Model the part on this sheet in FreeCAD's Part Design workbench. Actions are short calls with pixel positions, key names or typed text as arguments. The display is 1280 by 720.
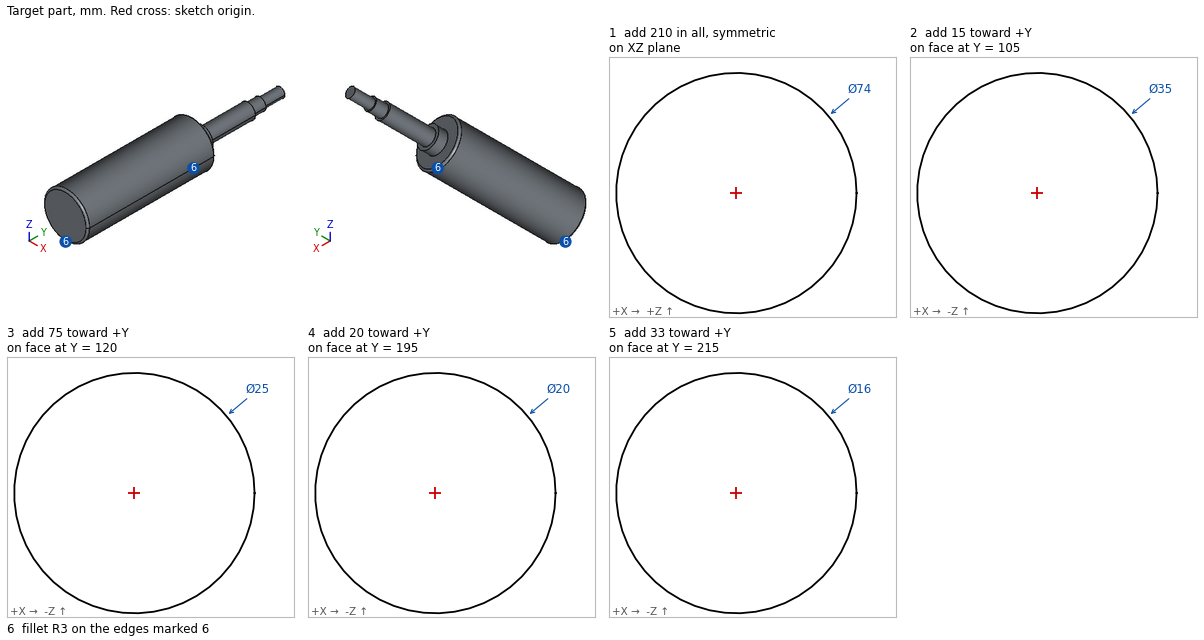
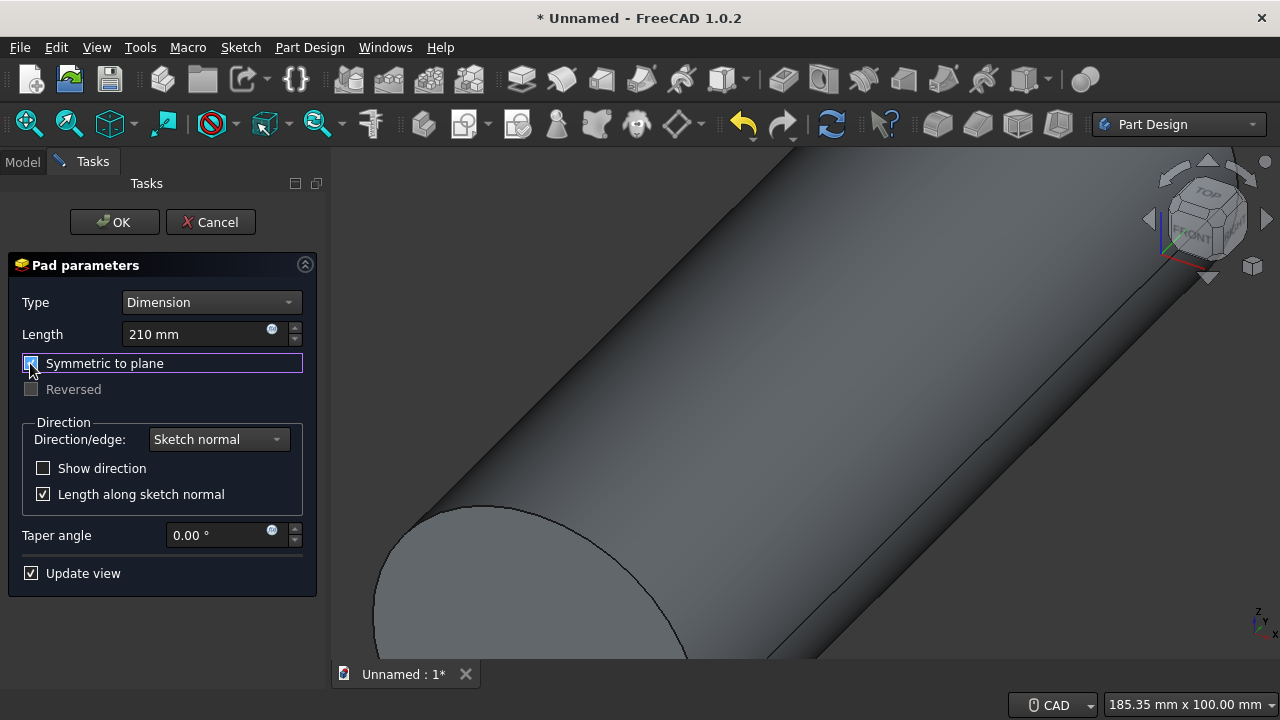
click(115, 222)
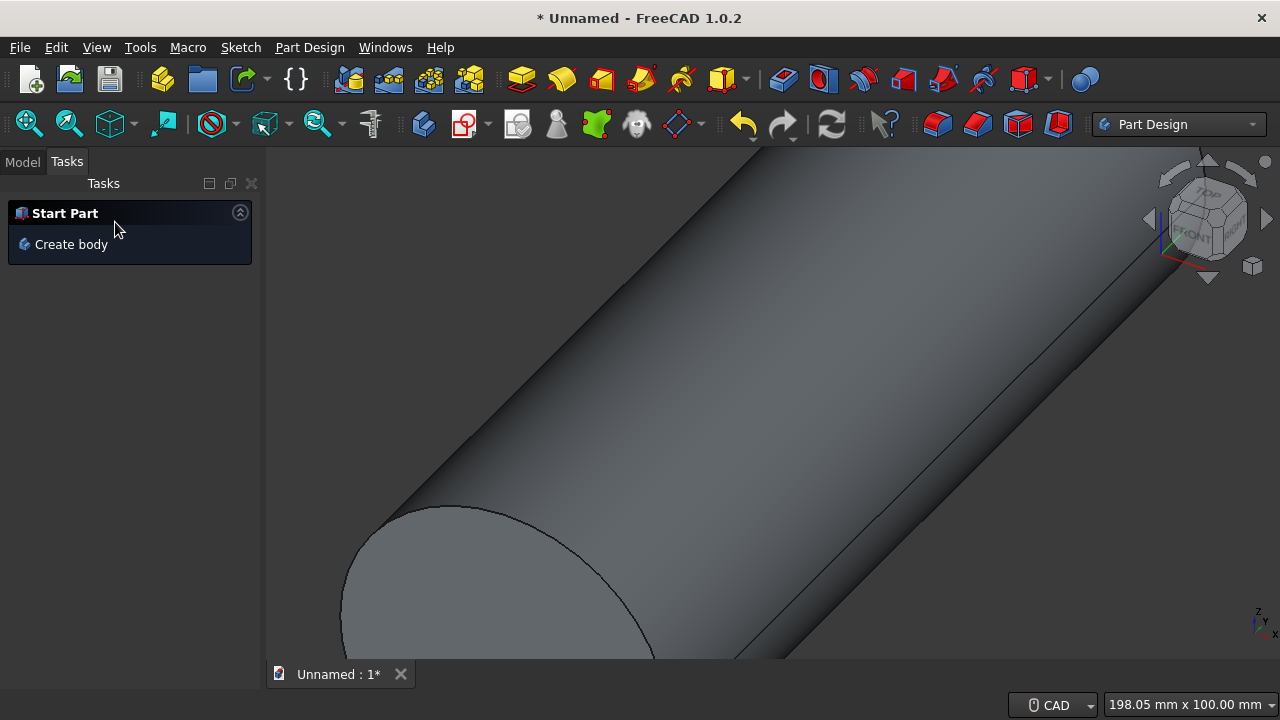
click(30, 124)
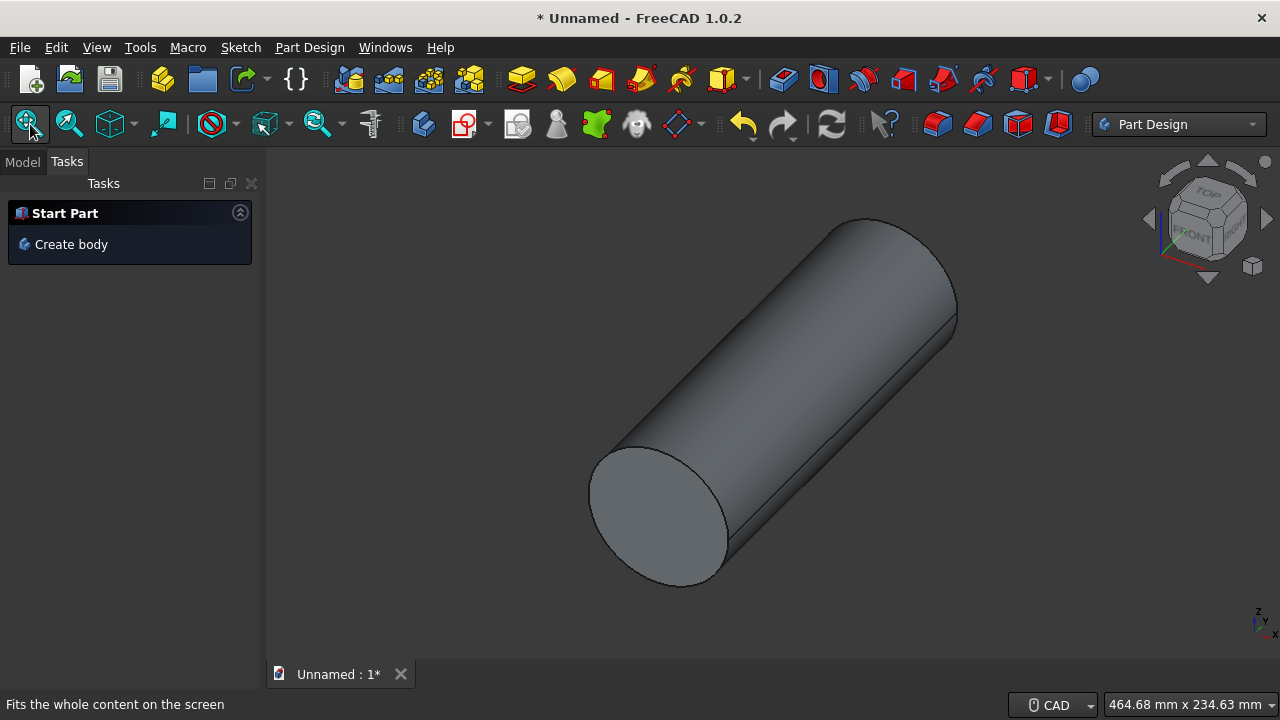
key(4)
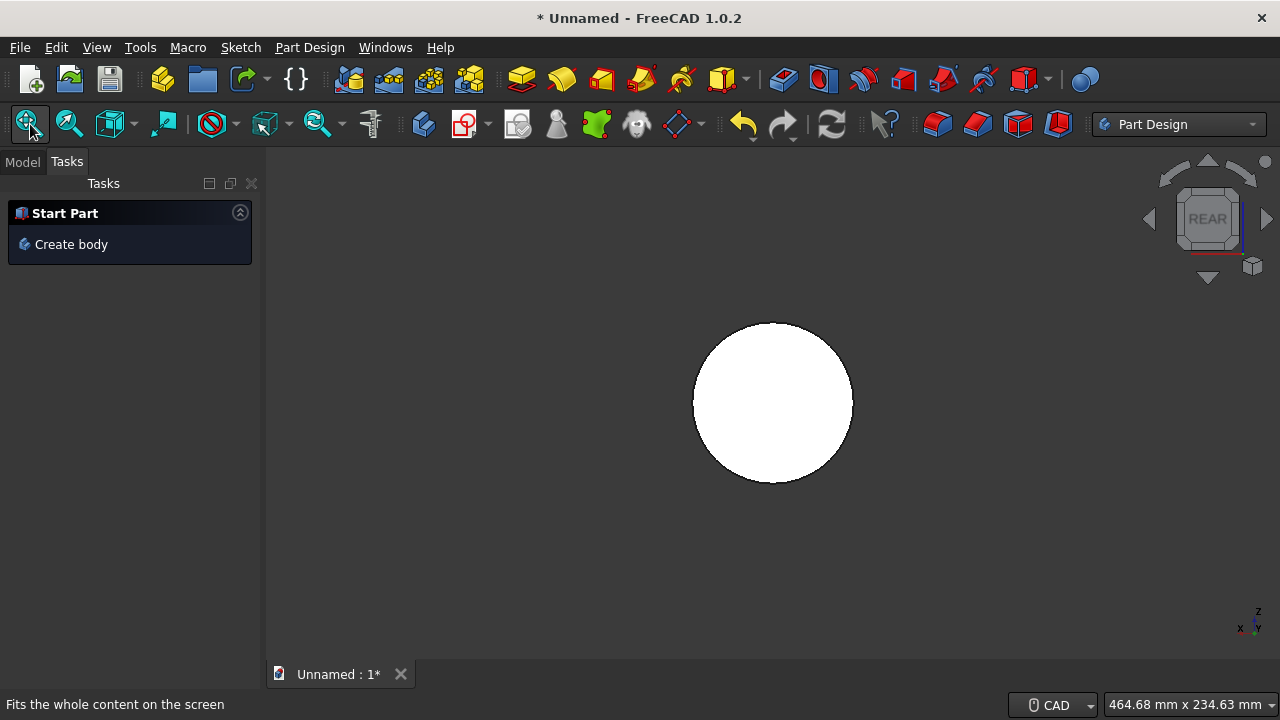
click(30, 124)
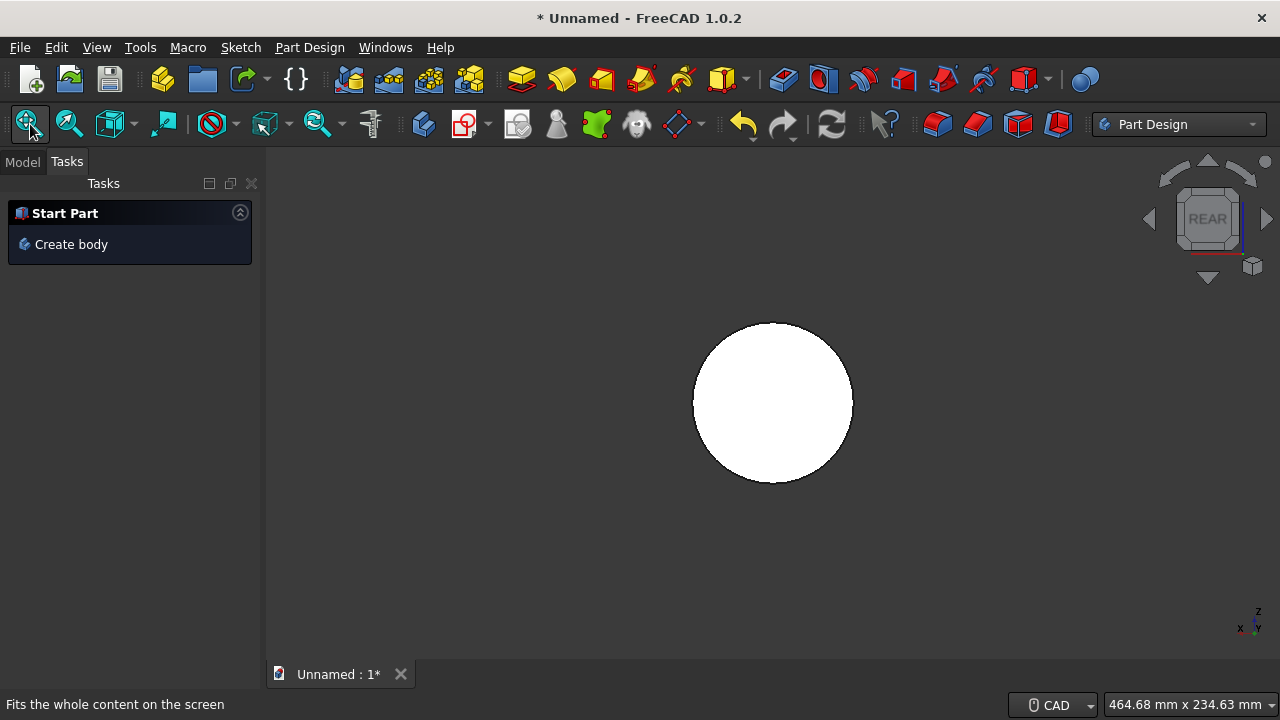
click(773, 402)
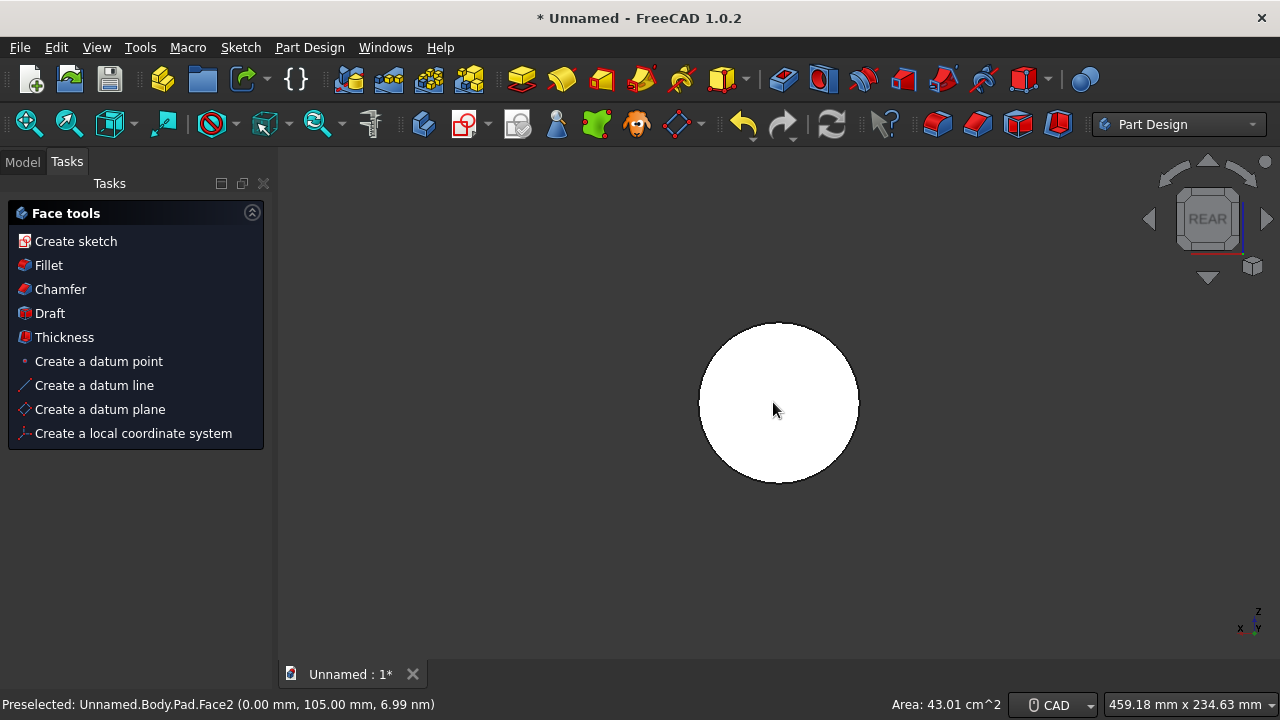
click(464, 124)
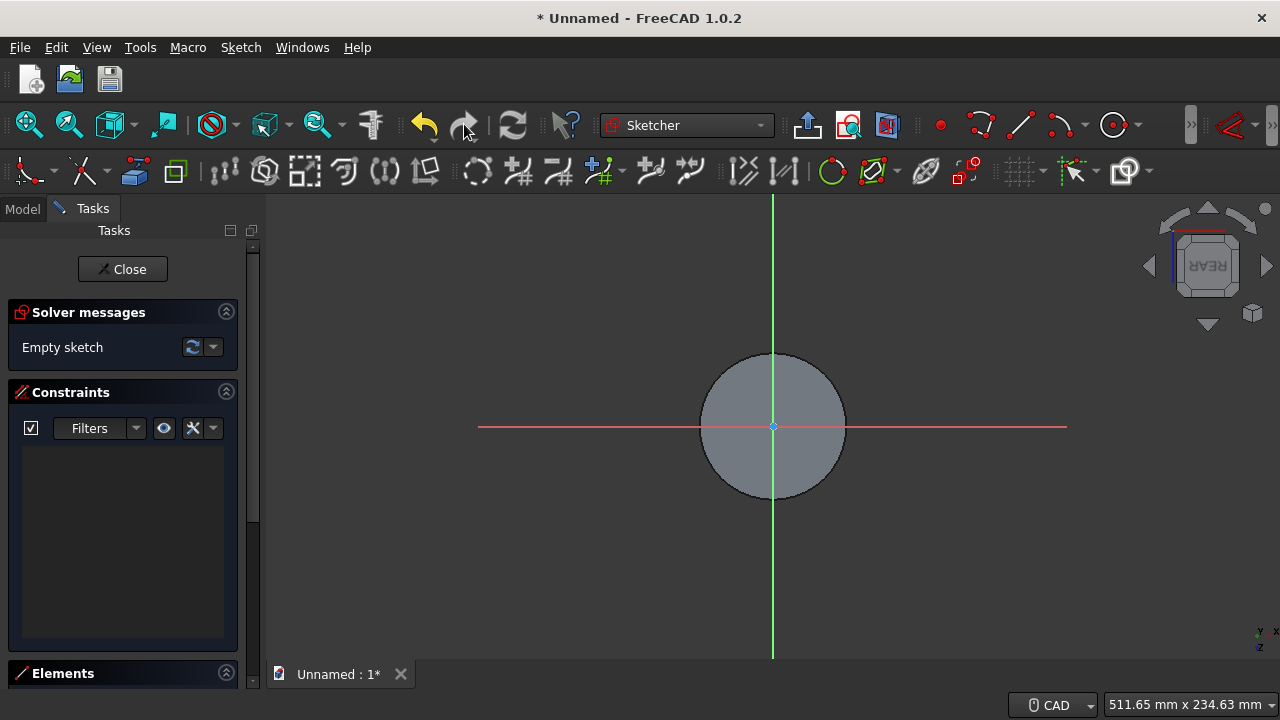
scroll(795, 426, up, 7)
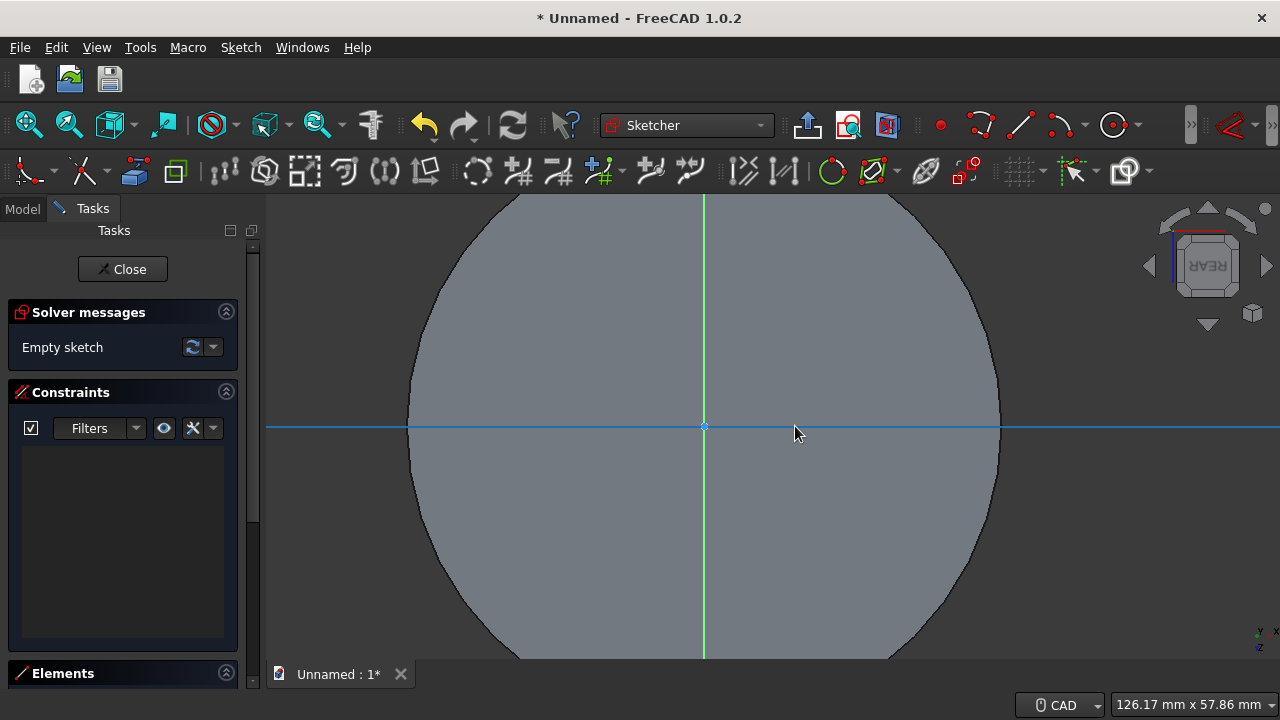
click(1114, 126)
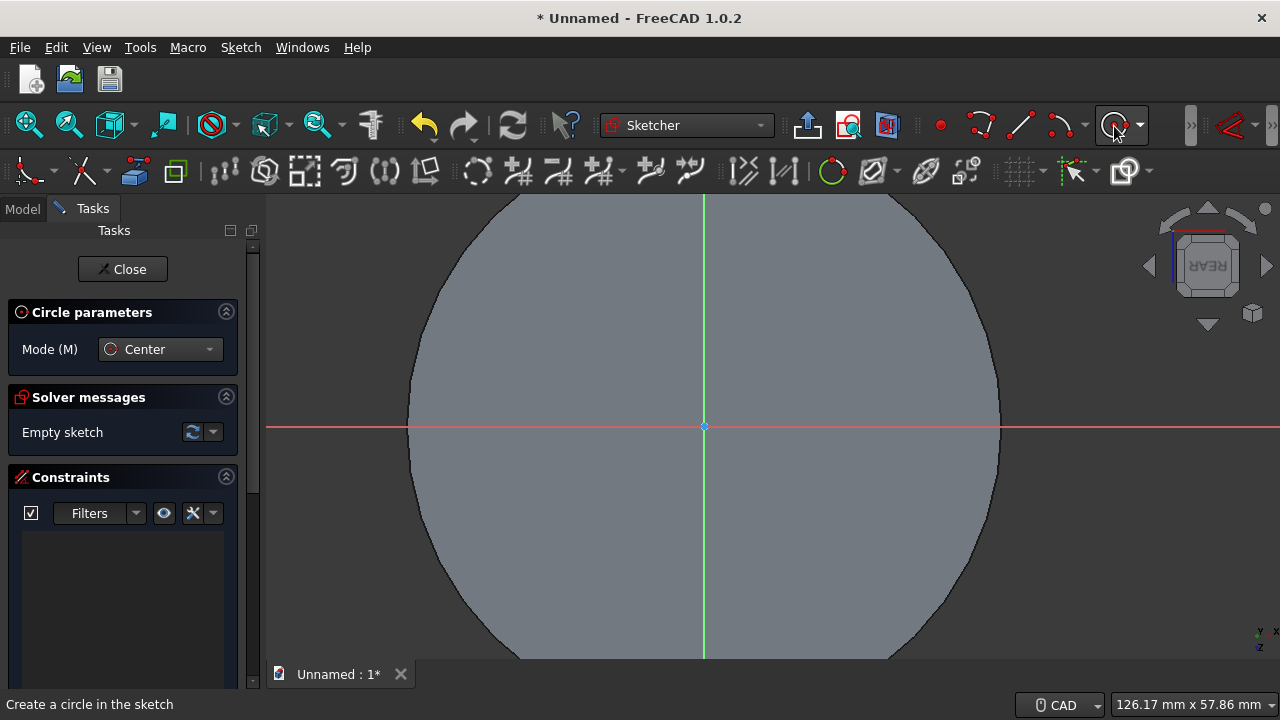
click(704, 426)
move(804, 327)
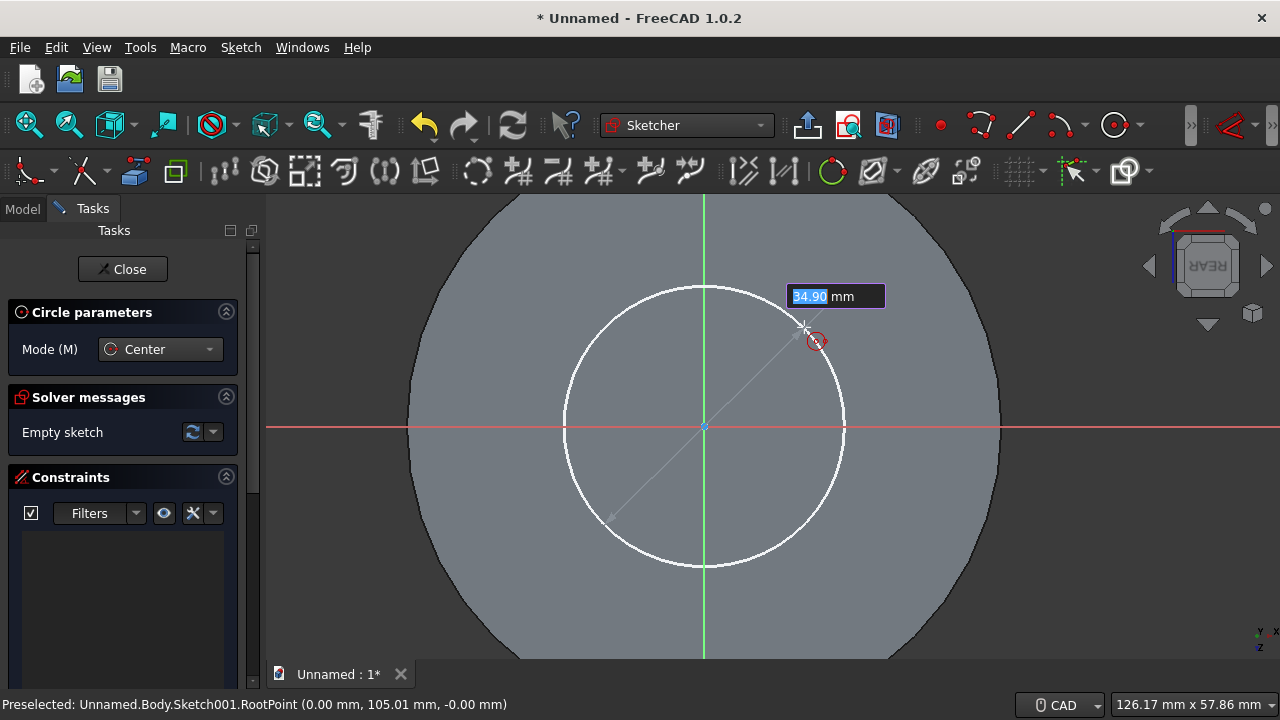
text(35)
key(Return)
key(Escape)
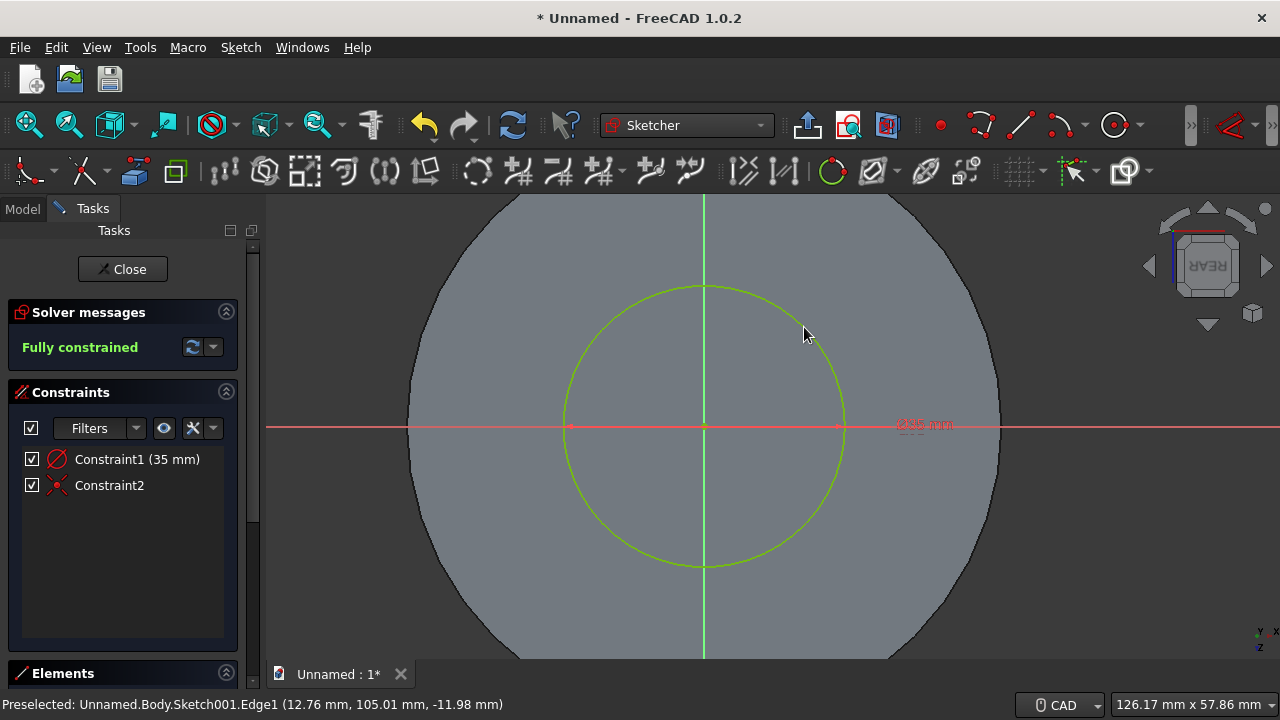
click(123, 269)